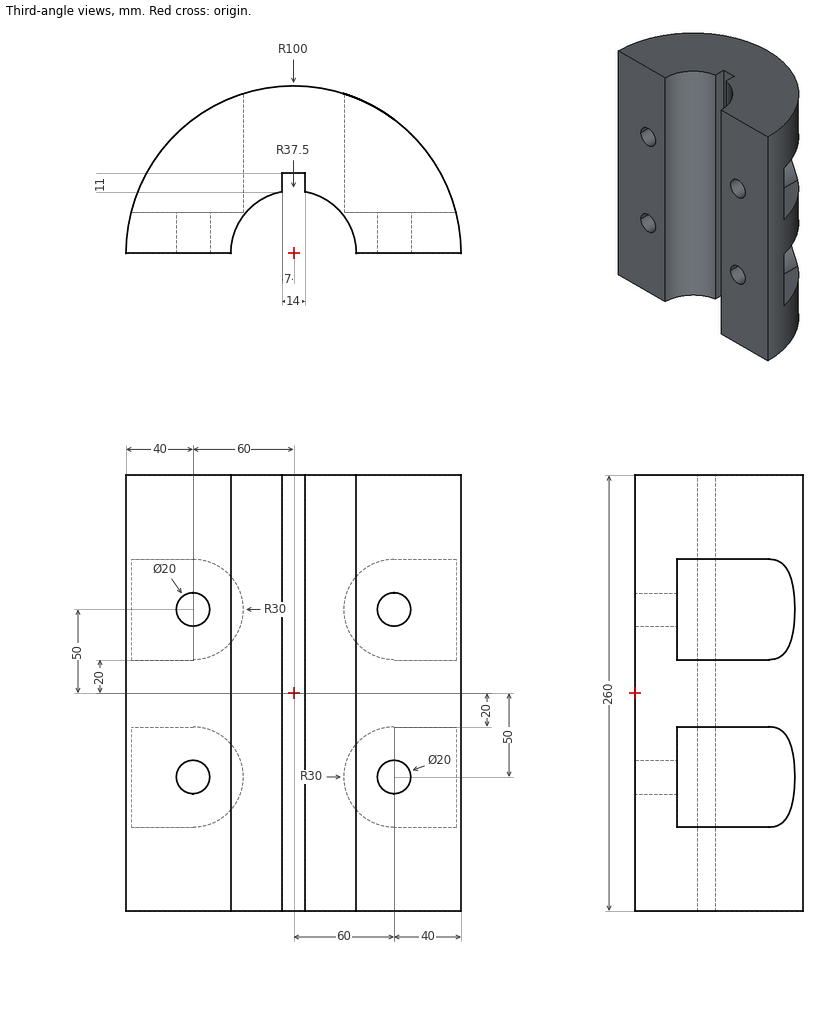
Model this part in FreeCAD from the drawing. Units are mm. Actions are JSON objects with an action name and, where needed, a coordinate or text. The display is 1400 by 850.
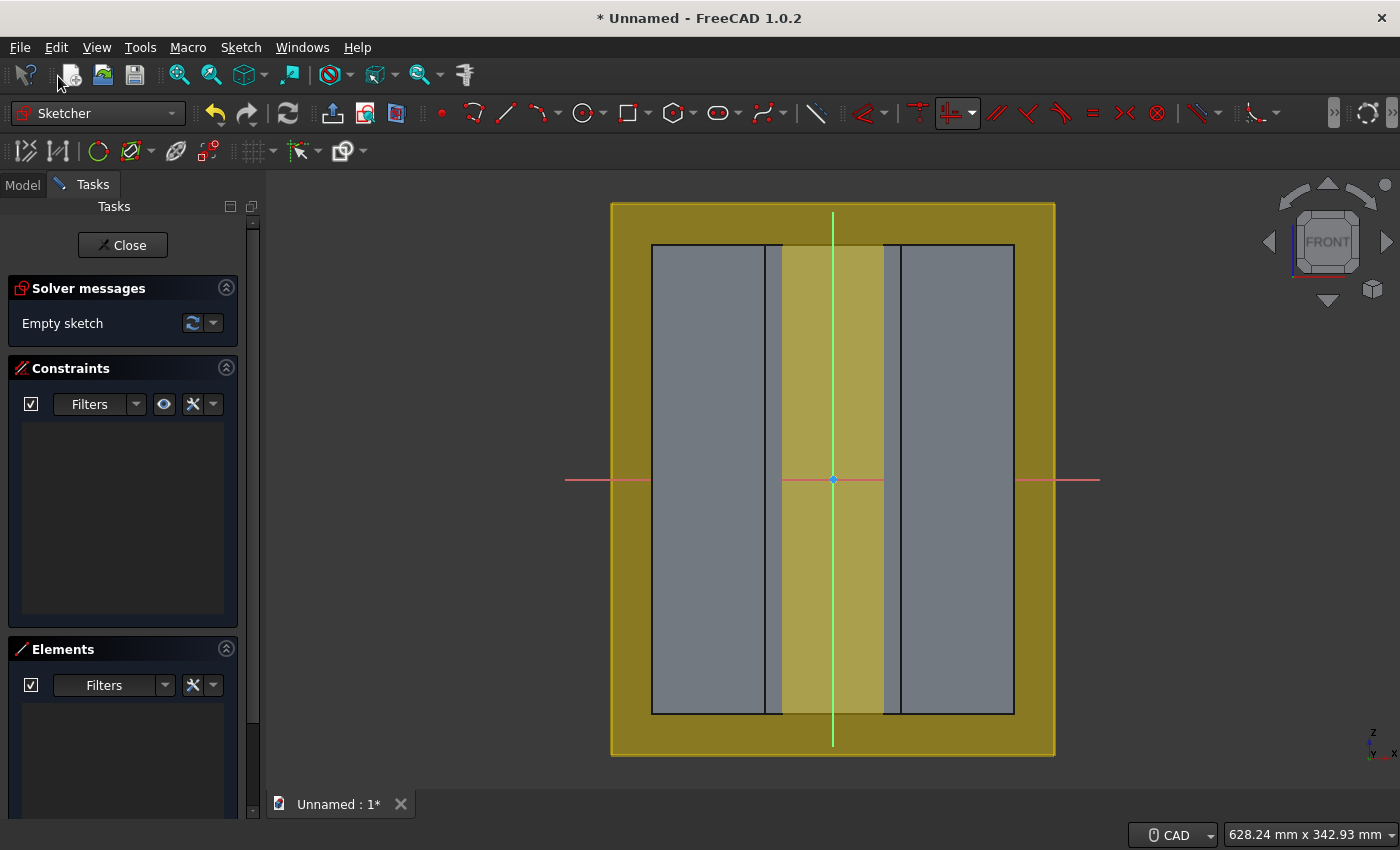
{"action": "left_click", "coordinate": [398, 114]}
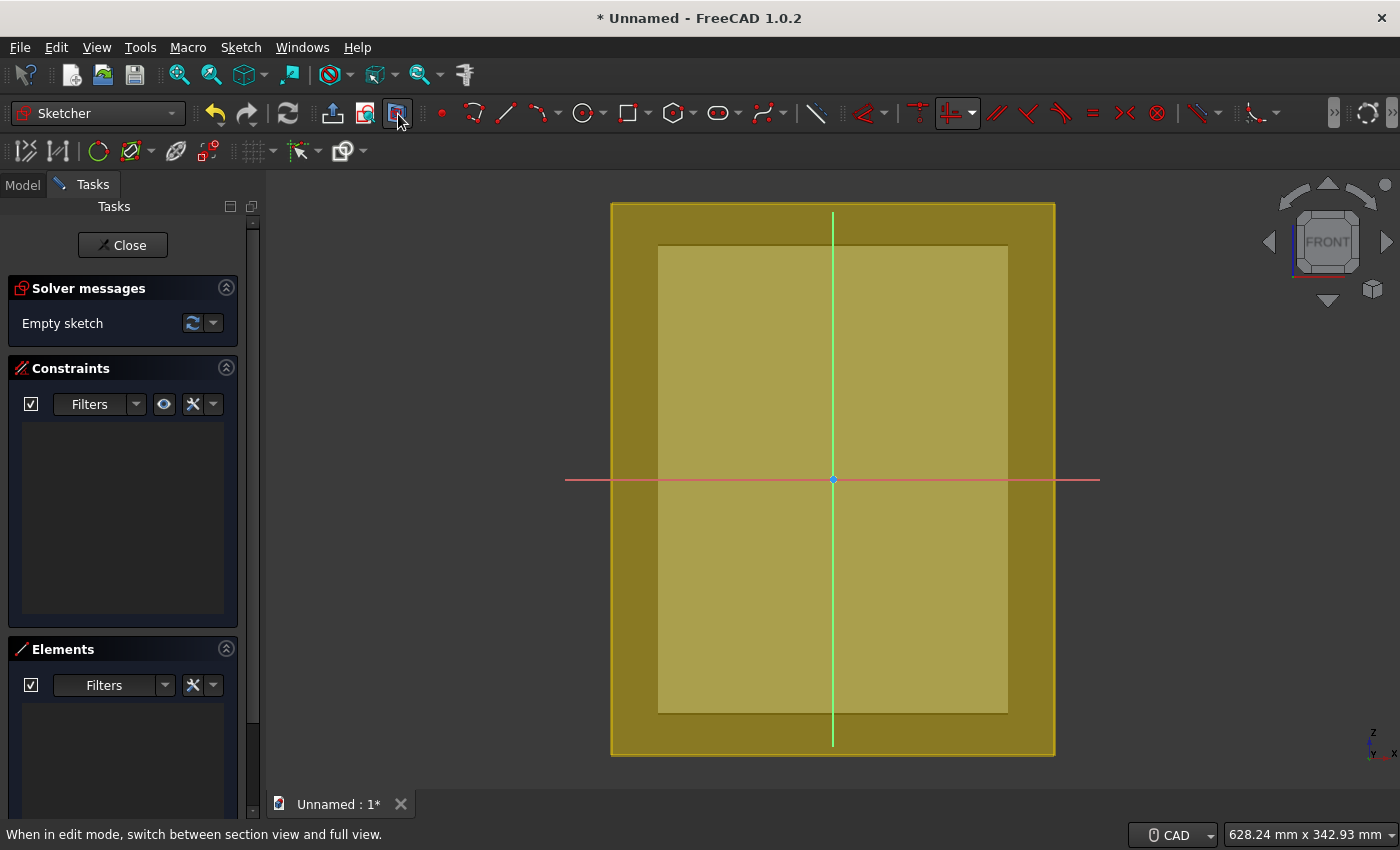
{"action": "scroll", "coordinate": [730, 365], "scroll_direction": "up", "scroll_amount": 5}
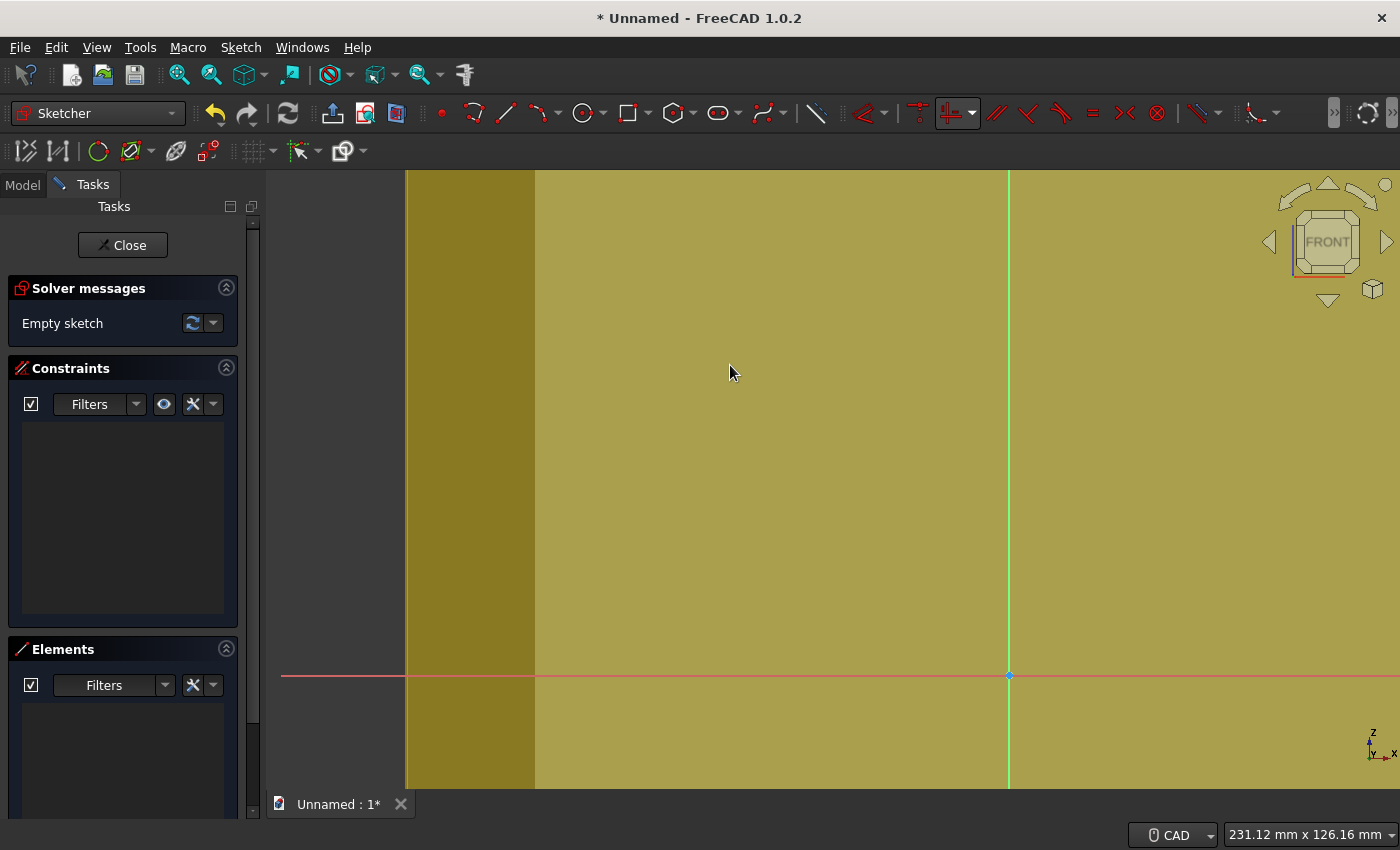
{"action": "left_click", "coordinate": [474, 114]}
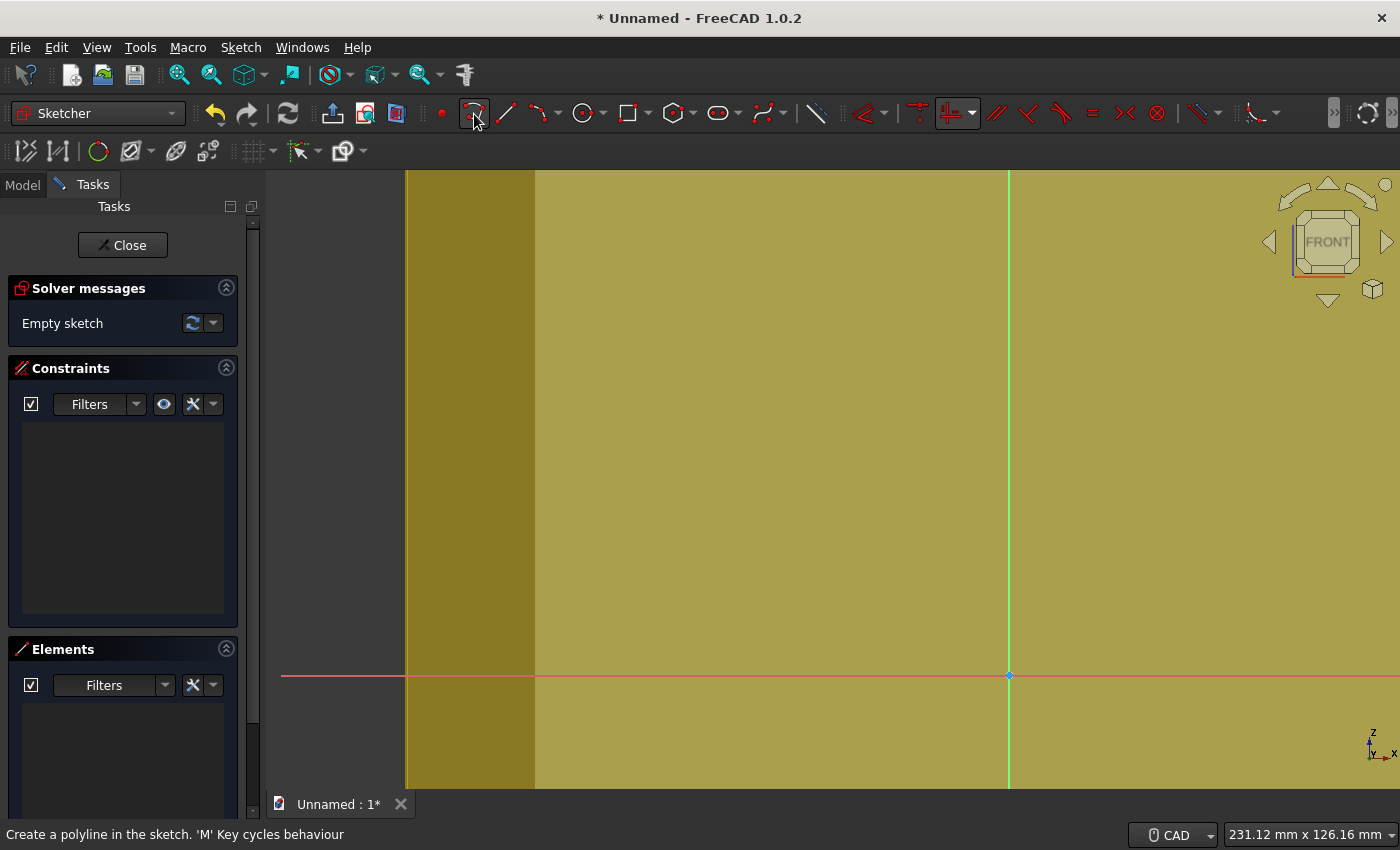
{"action": "left_click", "coordinate": [715, 578]}
{"action": "left_click", "coordinate": [519, 578]}
{"action": "left_click", "coordinate": [519, 283]}
{"action": "left_click", "coordinate": [715, 283]}
{"action": "right_click", "coordinate": [715, 283]}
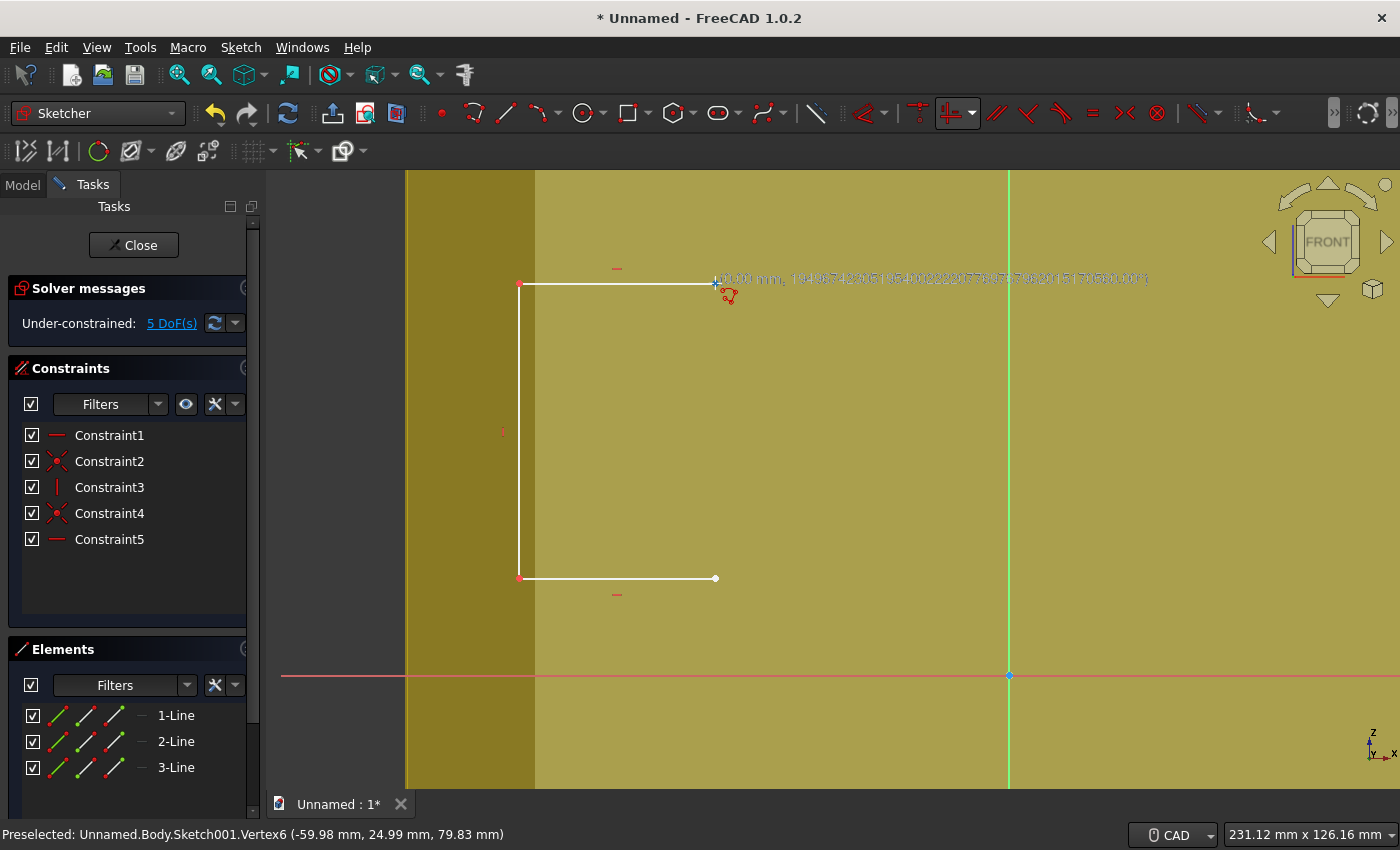
{"action": "left_click", "coordinate": [538, 114]}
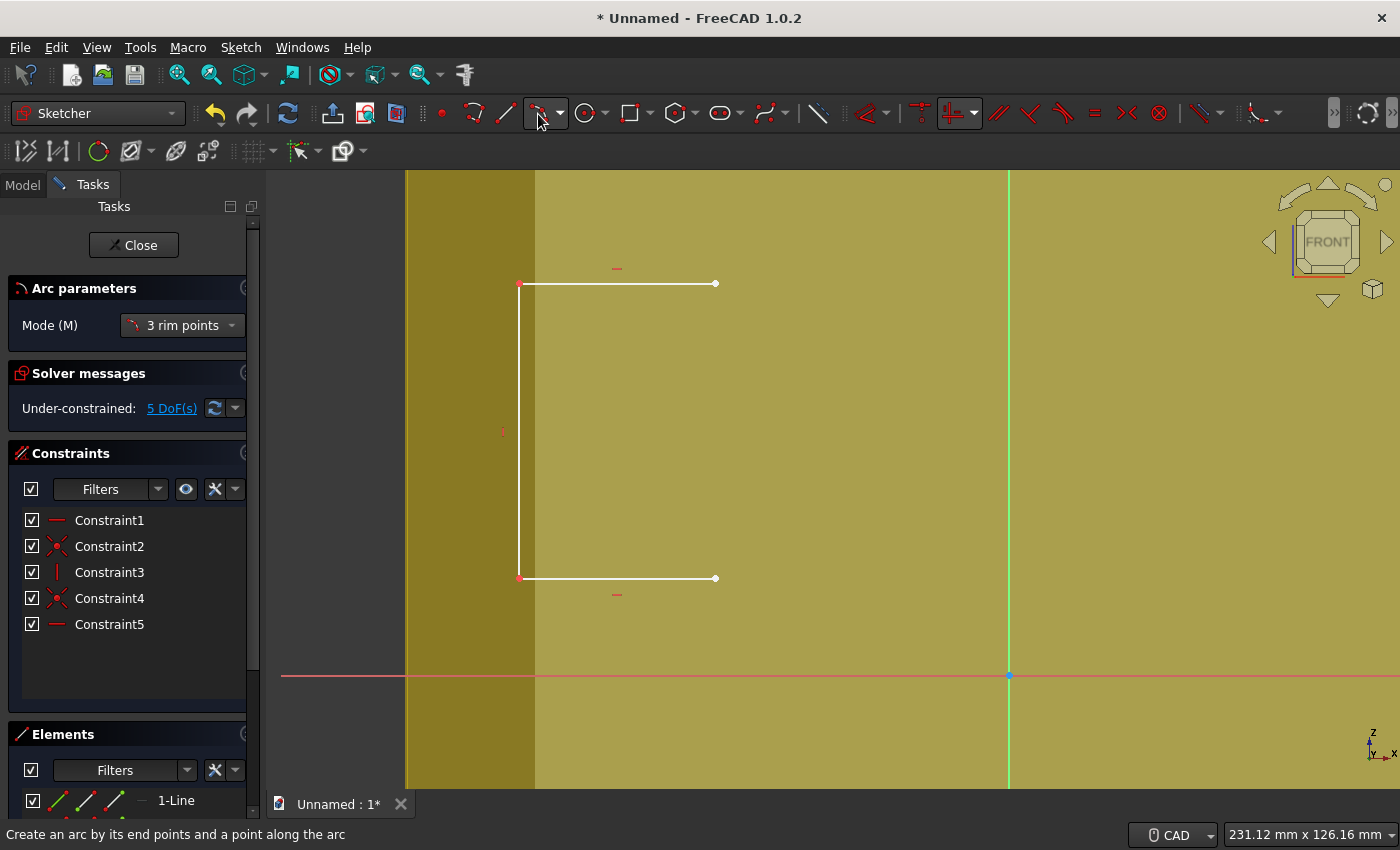
{"action": "left_click", "coordinate": [715, 284]}
{"action": "left_click", "coordinate": [715, 579]}
{"action": "left_click", "coordinate": [862, 430]}
{"action": "key", "text": "Escape"}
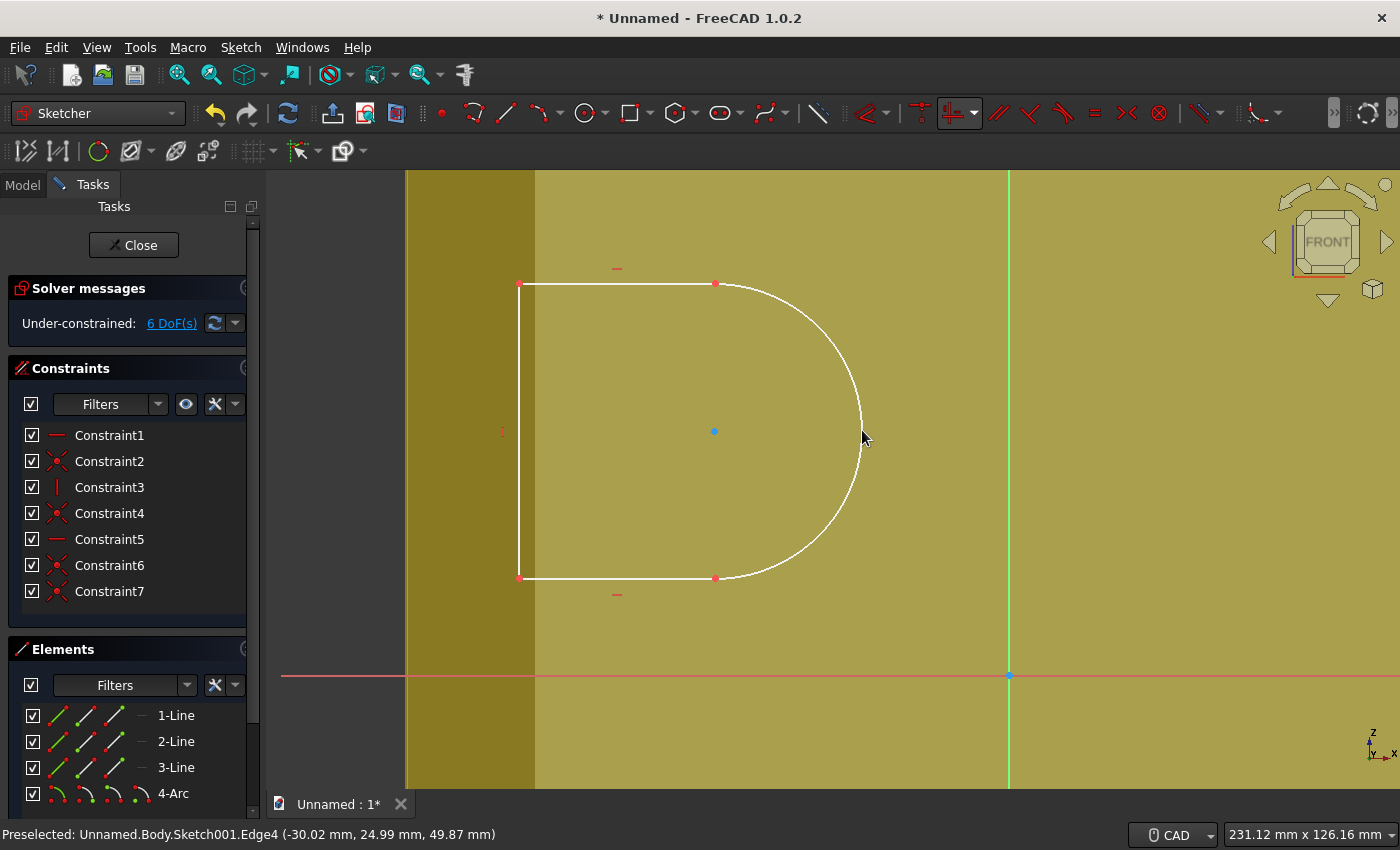
{"action": "left_click", "coordinate": [656, 579]}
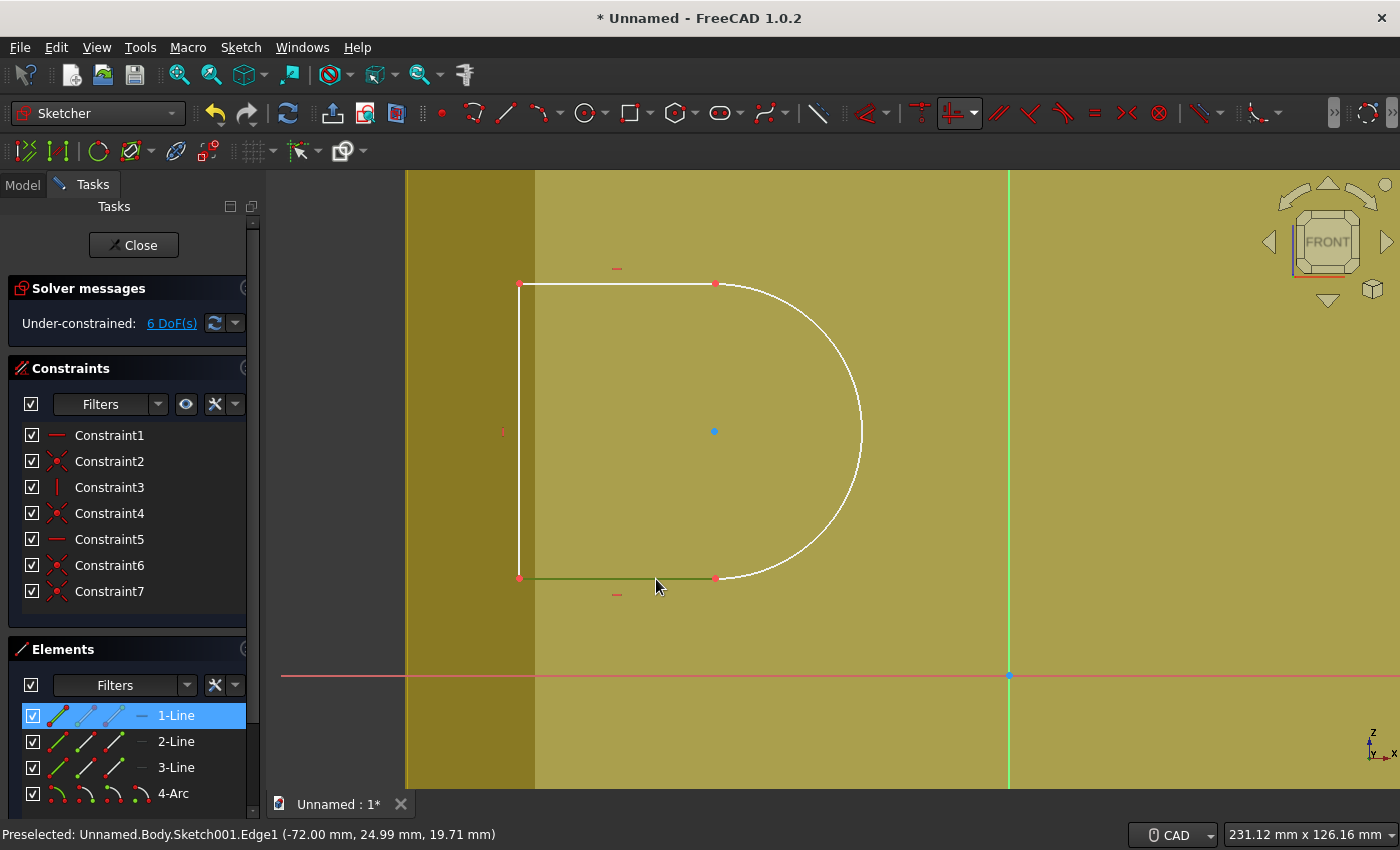
{"action": "left_click", "coordinate": [834, 518]}